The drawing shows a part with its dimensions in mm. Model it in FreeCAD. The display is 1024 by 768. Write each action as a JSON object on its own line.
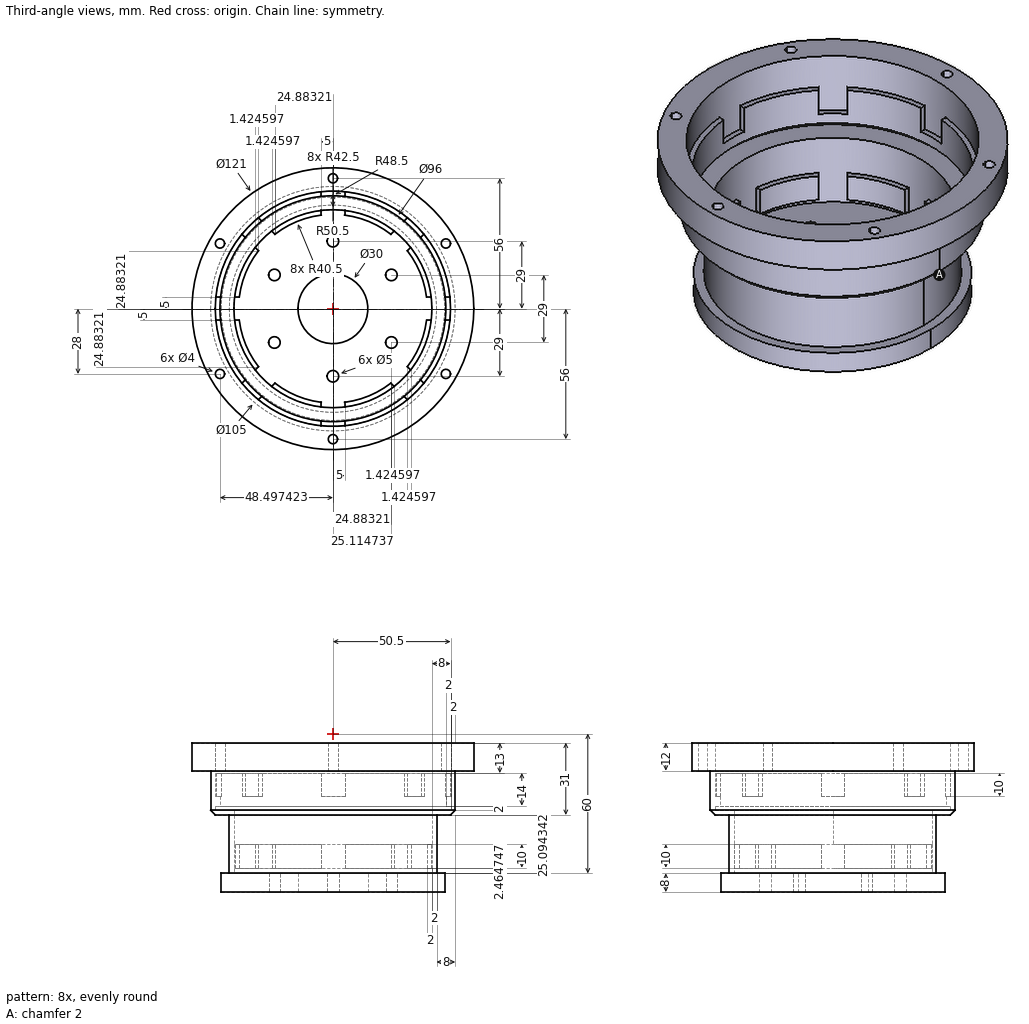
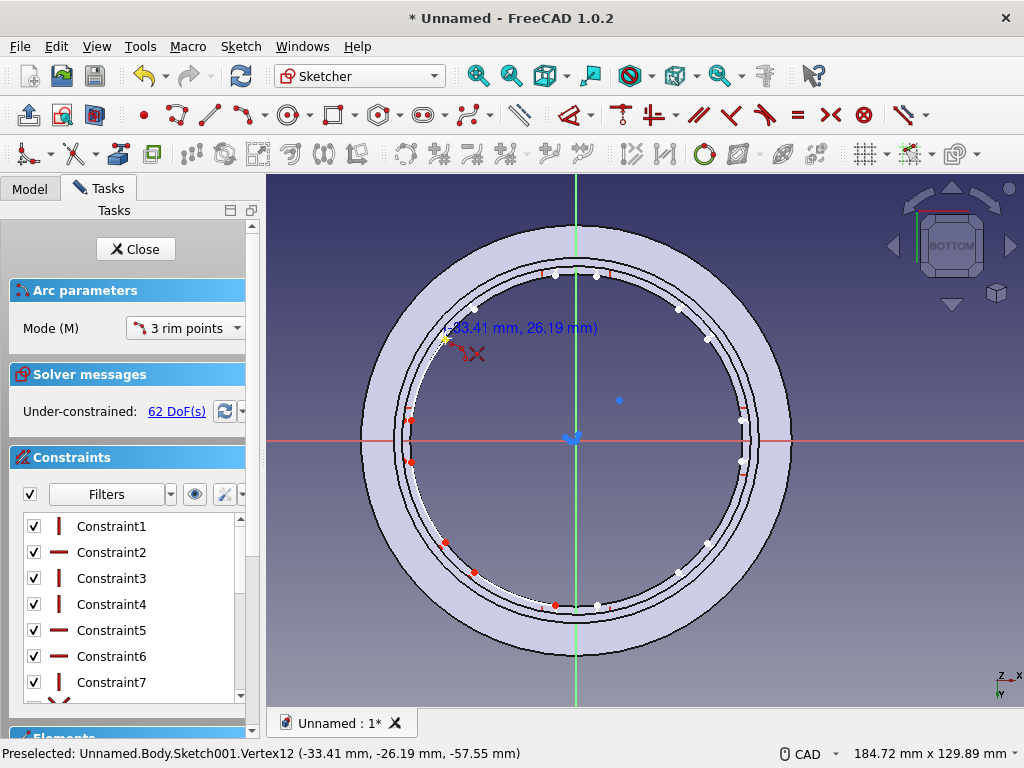
{"action": "scroll", "coordinate": [468, 304], "scroll_direction": "up", "scroll_amount": 7}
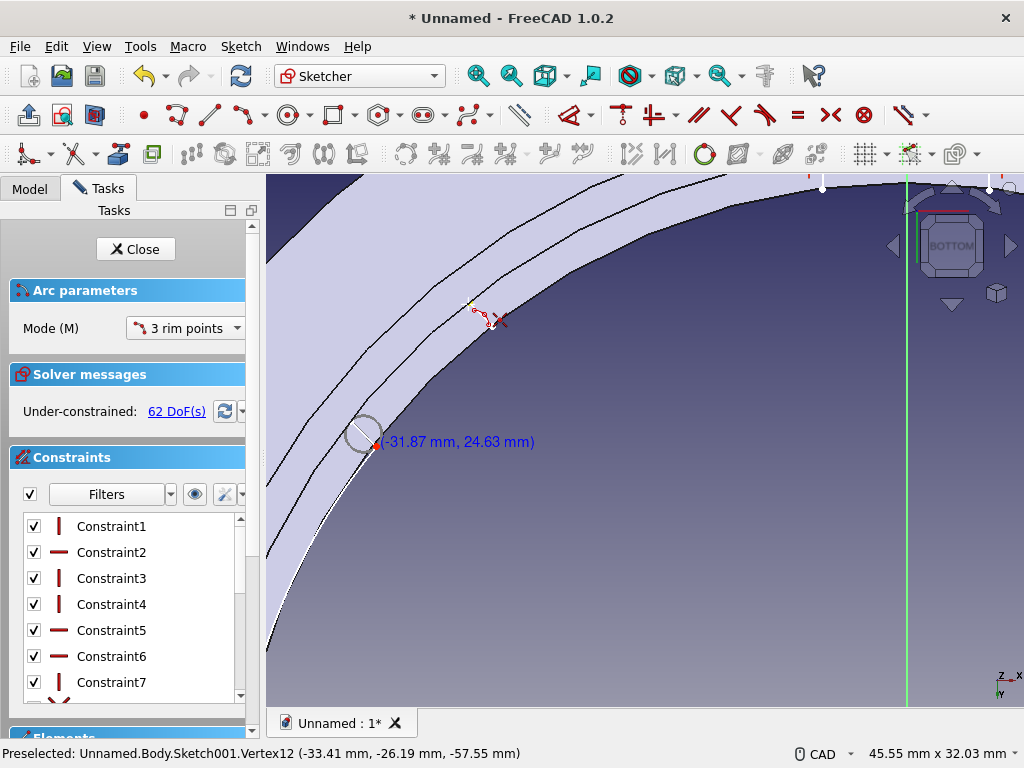
{"action": "left_click", "coordinate": [469, 303]}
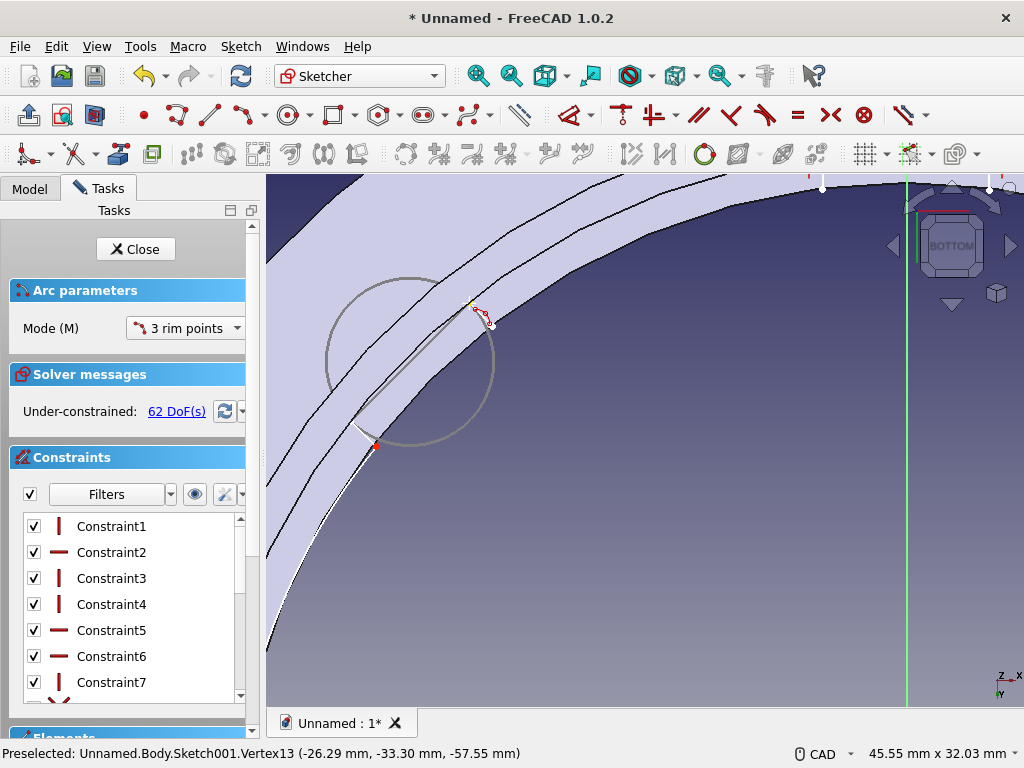
{"action": "scroll", "coordinate": [407, 357], "scroll_direction": "up", "scroll_amount": 6}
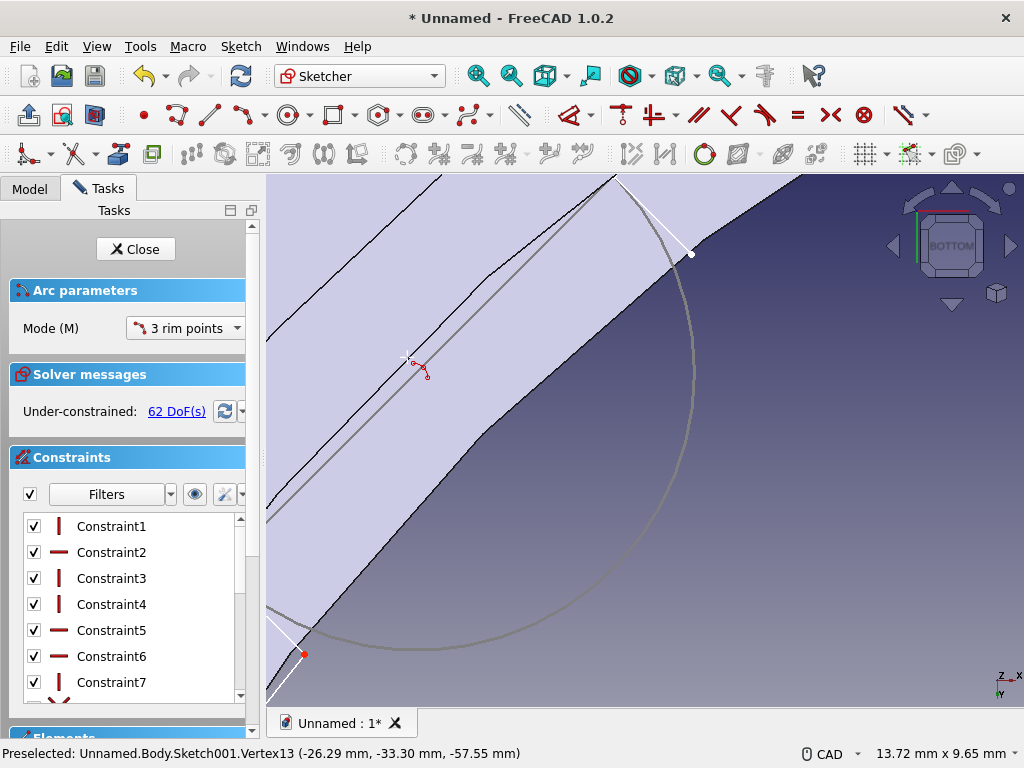
{"action": "left_click", "coordinate": [405, 355]}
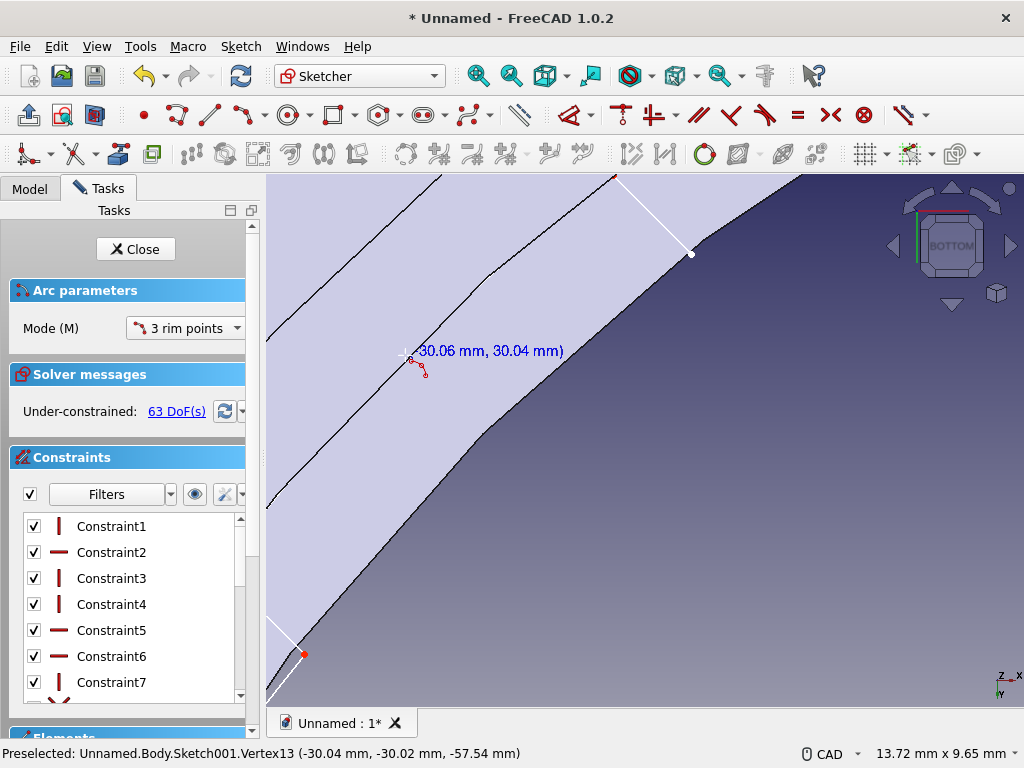
{"action": "scroll", "coordinate": [457, 314], "scroll_direction": "down", "scroll_amount": 13}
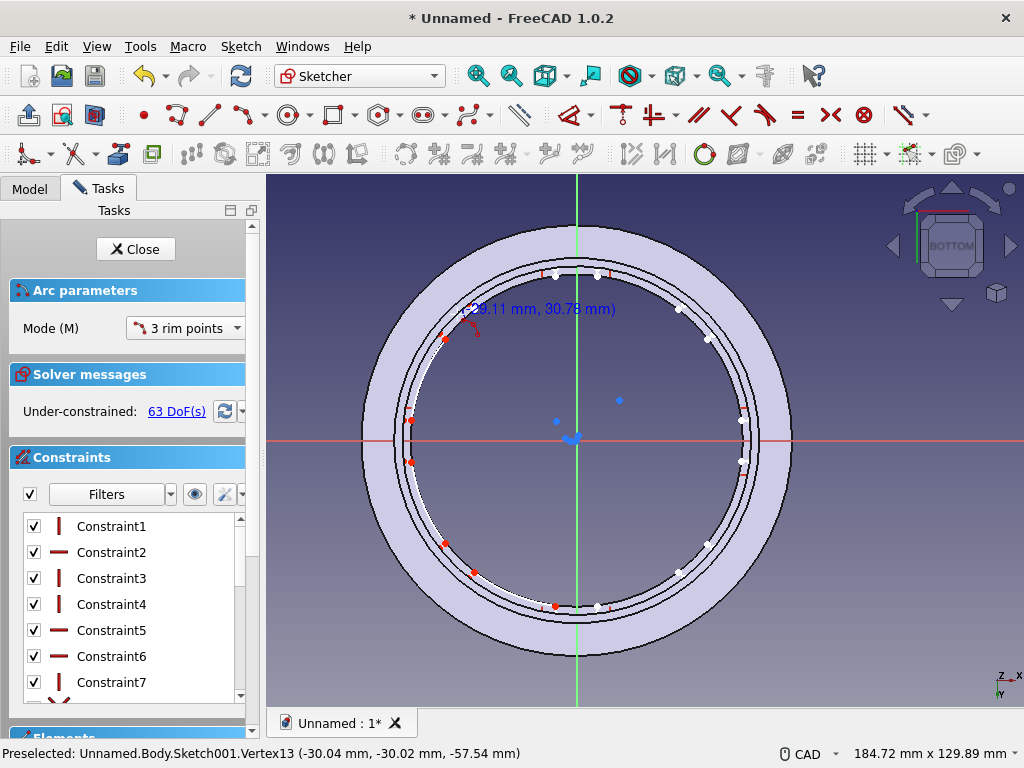
{"action": "scroll", "coordinate": [475, 310], "scroll_direction": "up", "scroll_amount": 7}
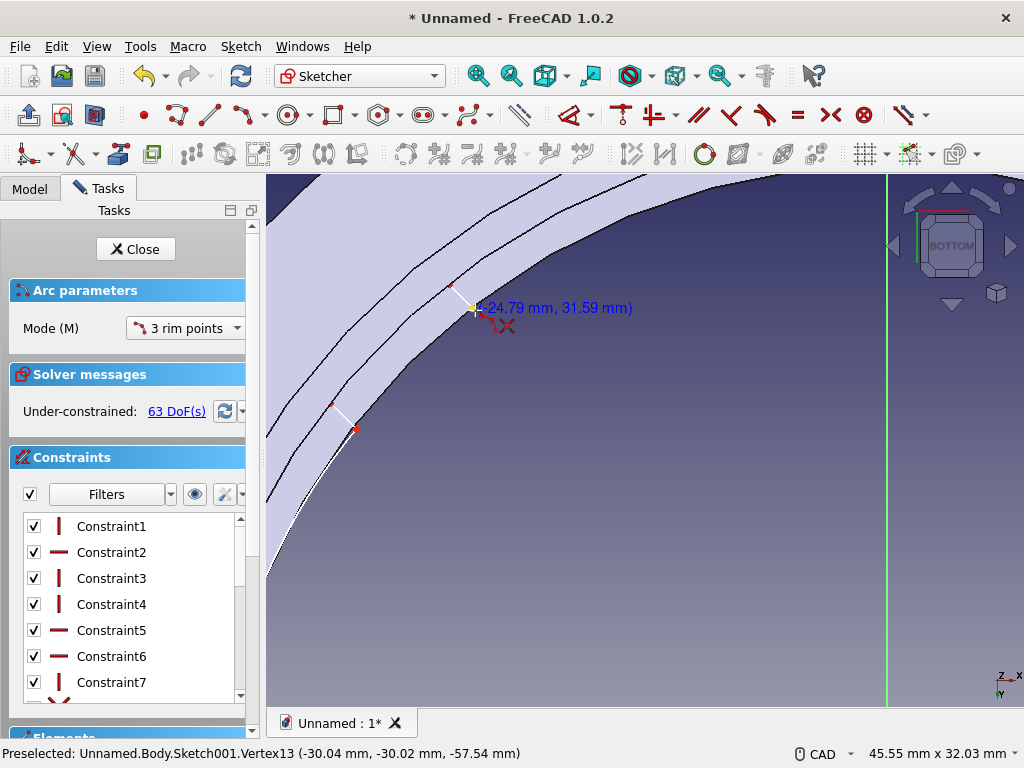
{"action": "left_click", "coordinate": [473, 308]}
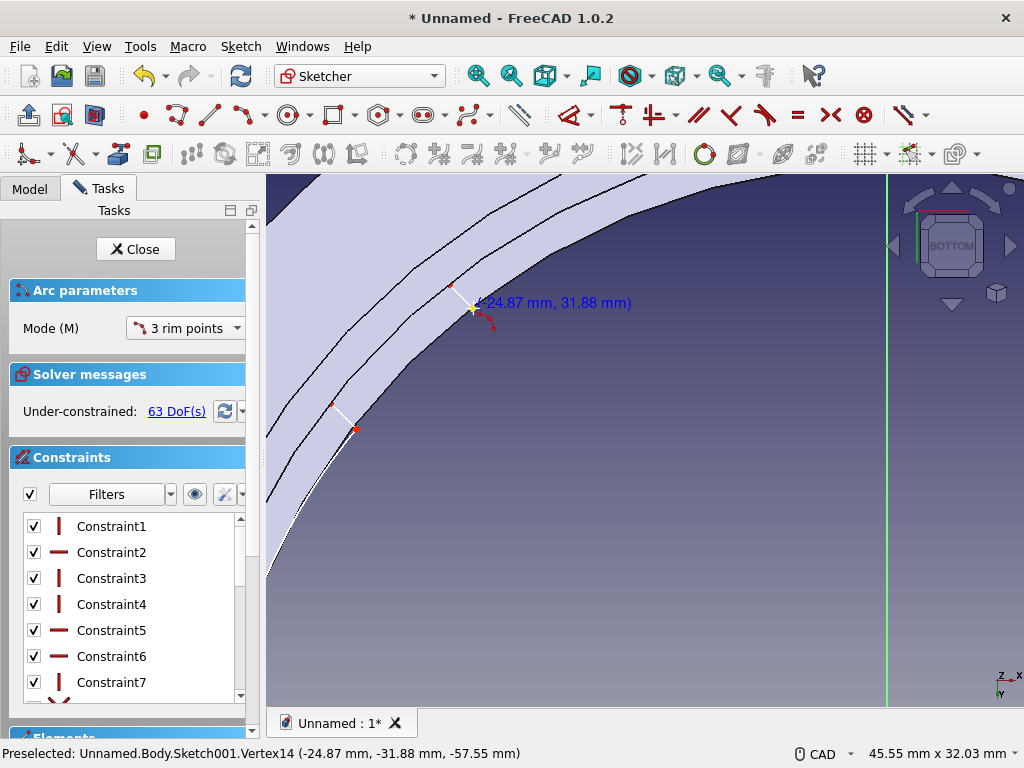
{"action": "scroll", "coordinate": [475, 310], "scroll_direction": "down", "scroll_amount": 7}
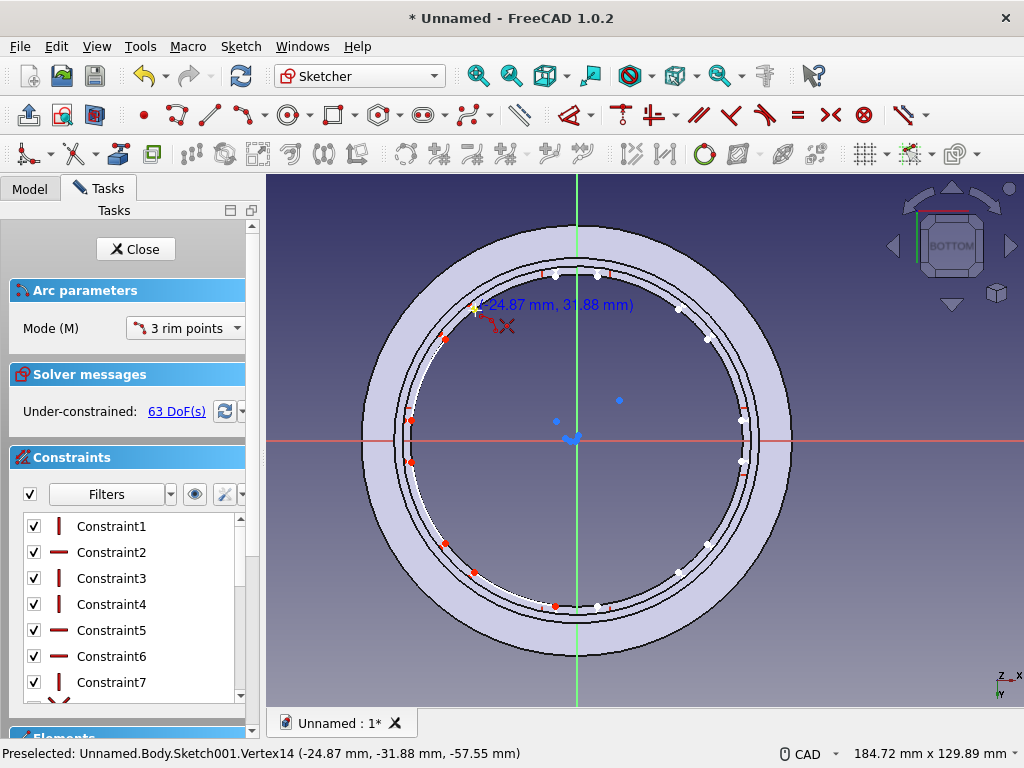
{"action": "scroll", "coordinate": [556, 276], "scroll_direction": "up", "scroll_amount": 7}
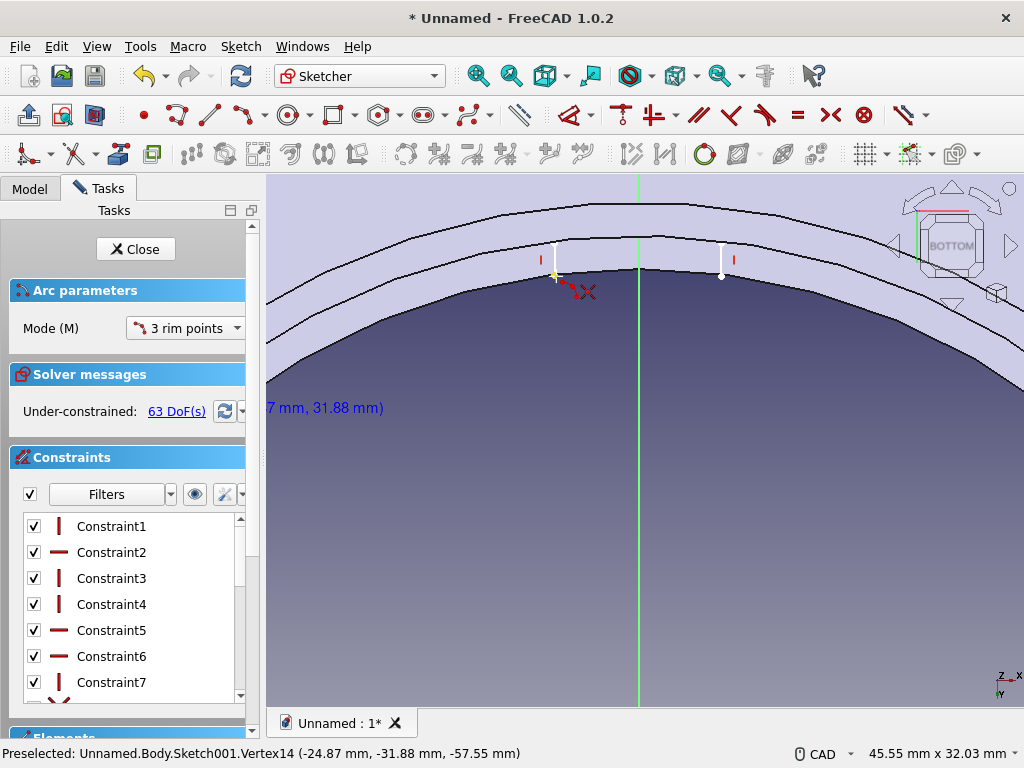
{"action": "left_click", "coordinate": [555, 276]}
{"action": "left_click", "coordinate": [381, 320]}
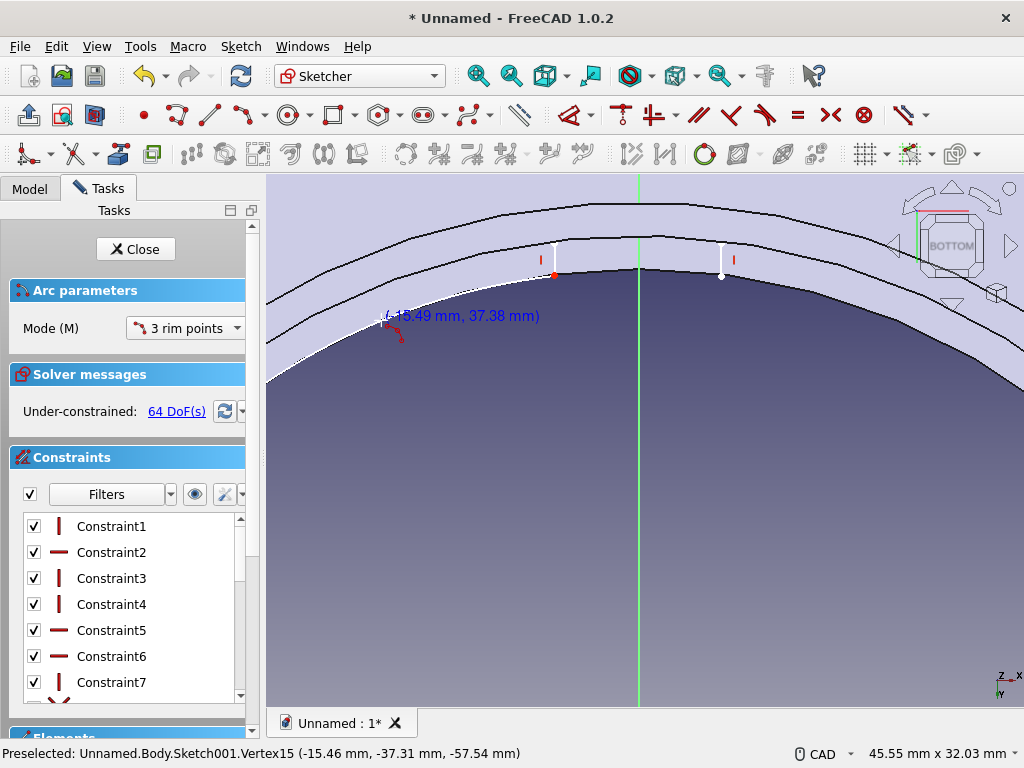
{"action": "left_click", "coordinate": [555, 243]}
{"action": "left_click", "coordinate": [721, 243]}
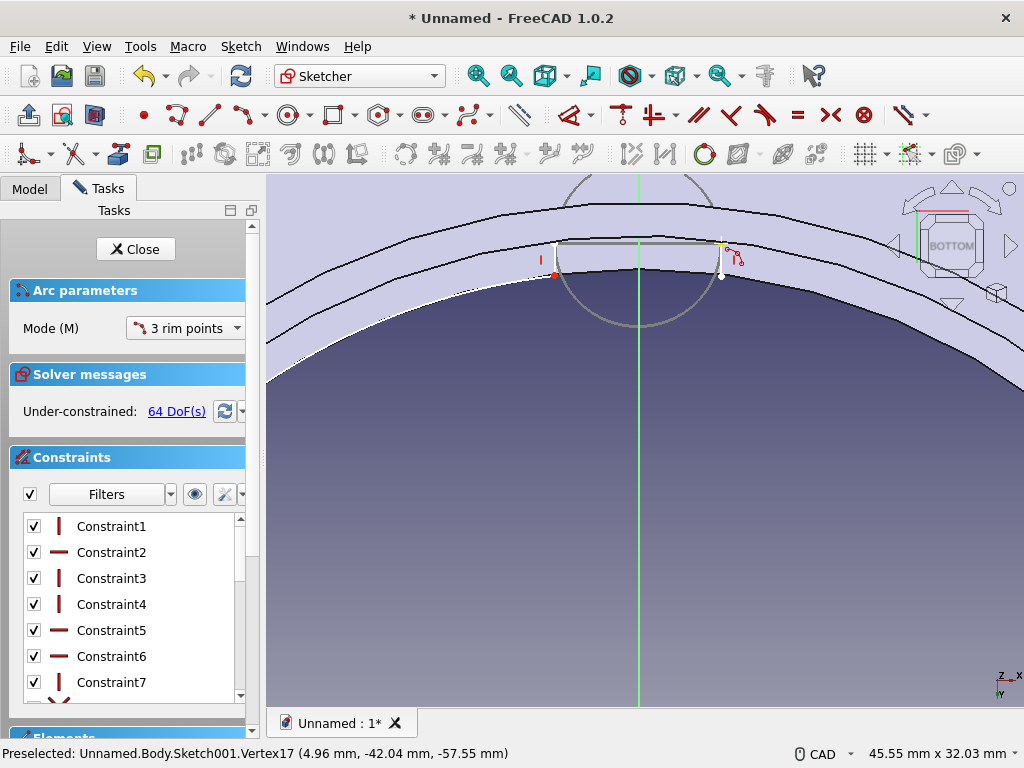
{"action": "scroll", "coordinate": [655, 236], "scroll_direction": "up", "scroll_amount": 7}